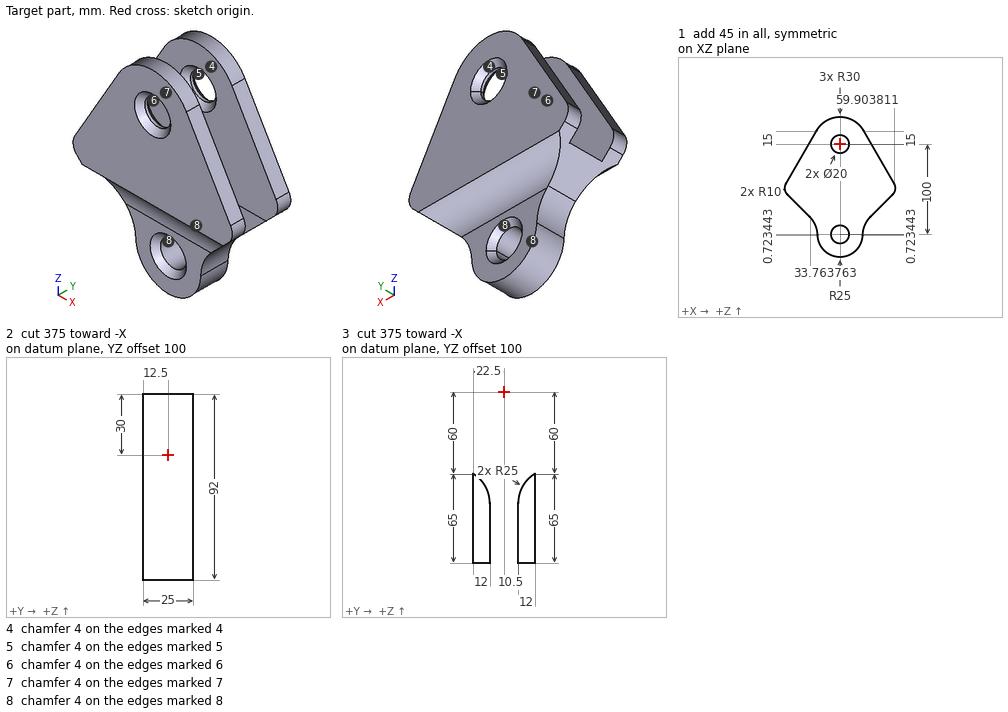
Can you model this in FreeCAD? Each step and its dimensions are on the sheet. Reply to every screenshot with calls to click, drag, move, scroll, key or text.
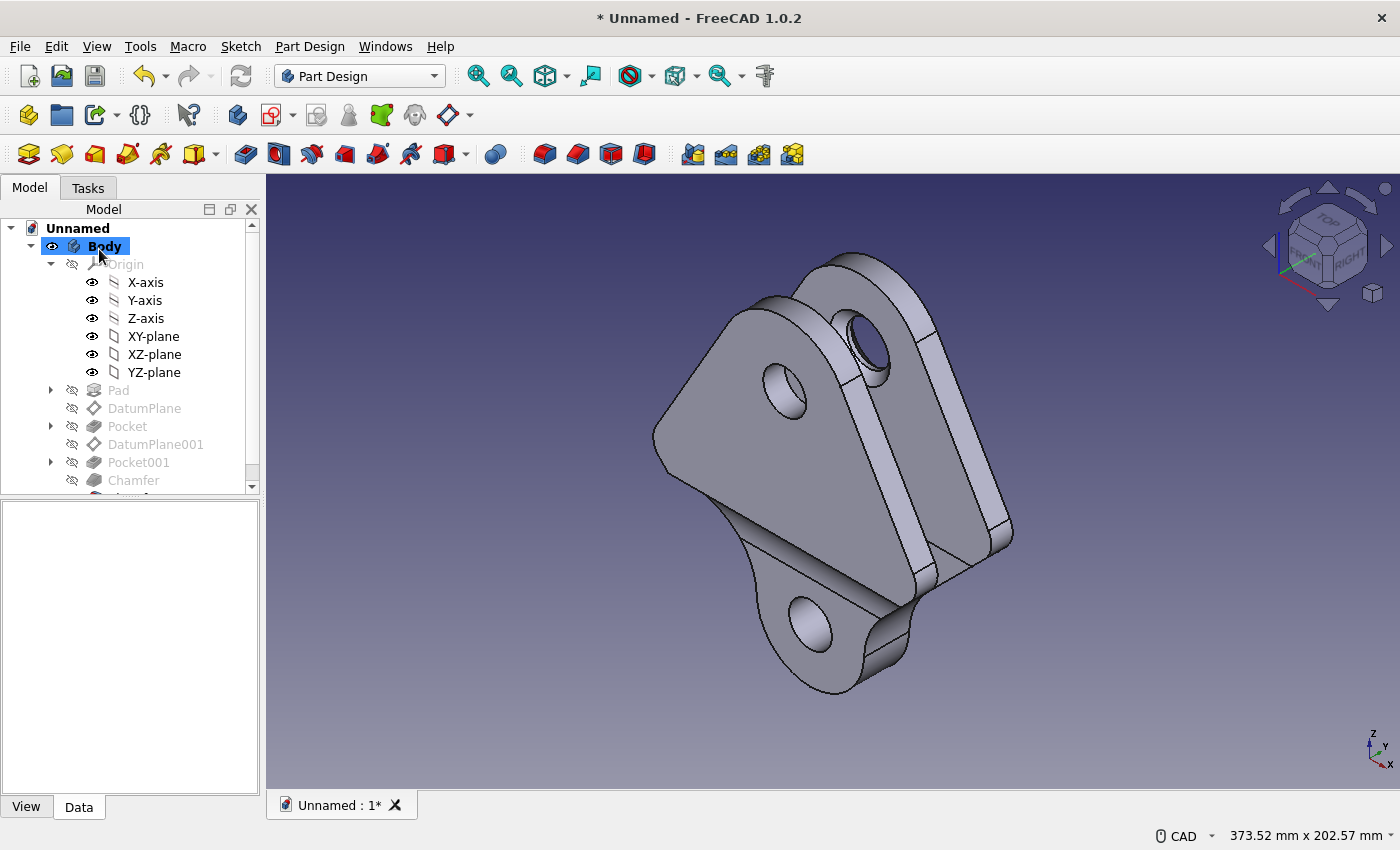
click(763, 378)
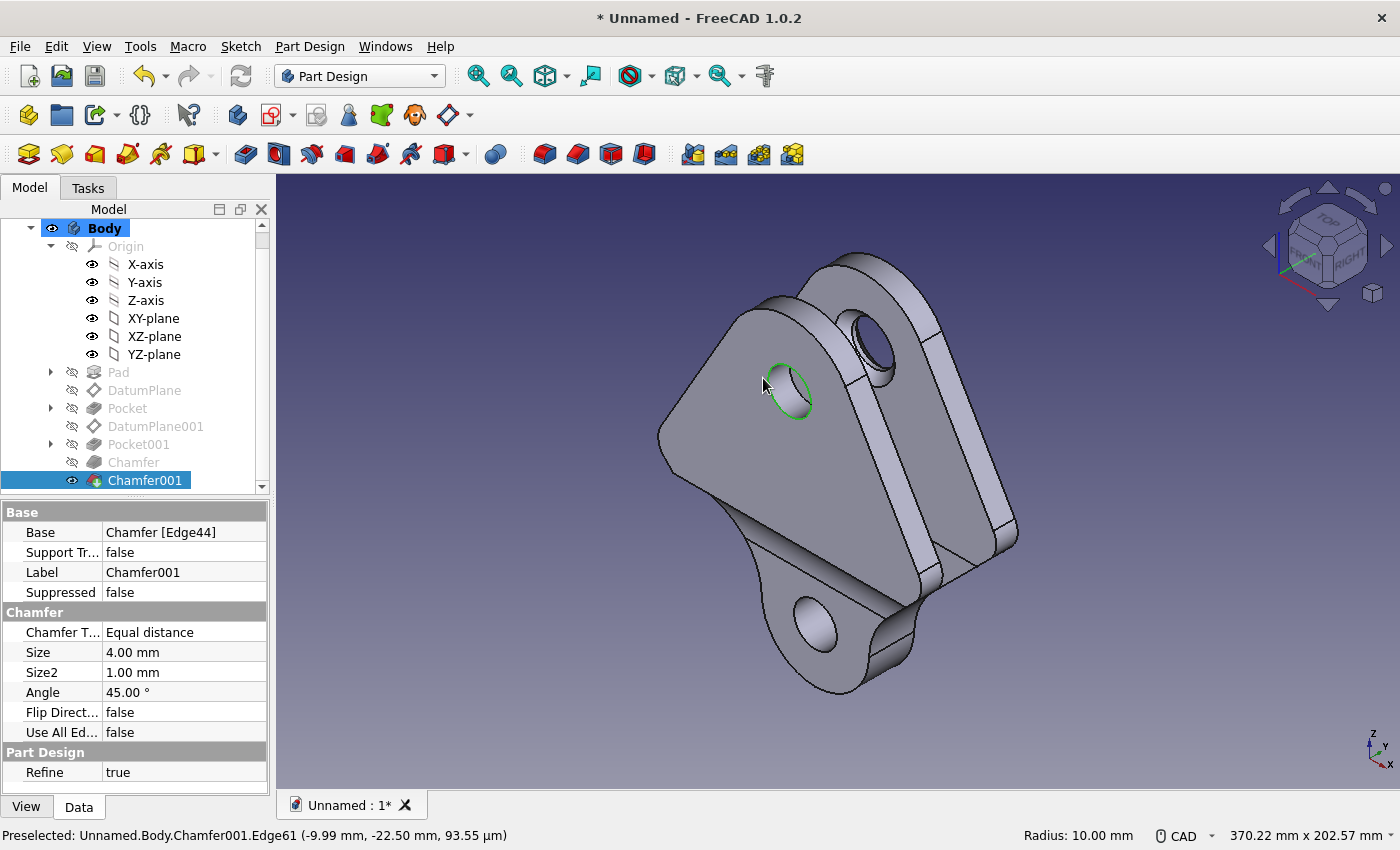
click(578, 154)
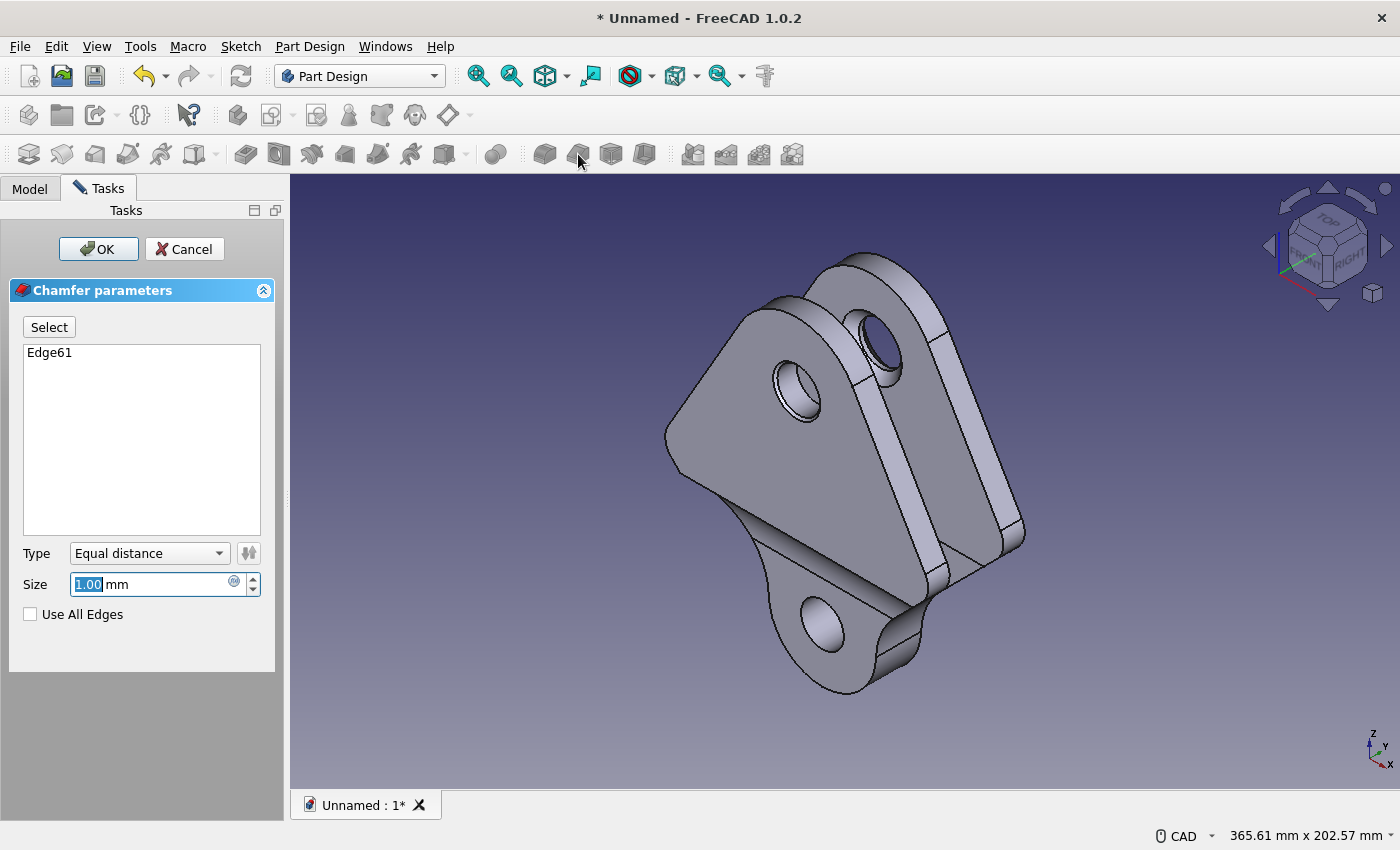
text(4)
key(Tab)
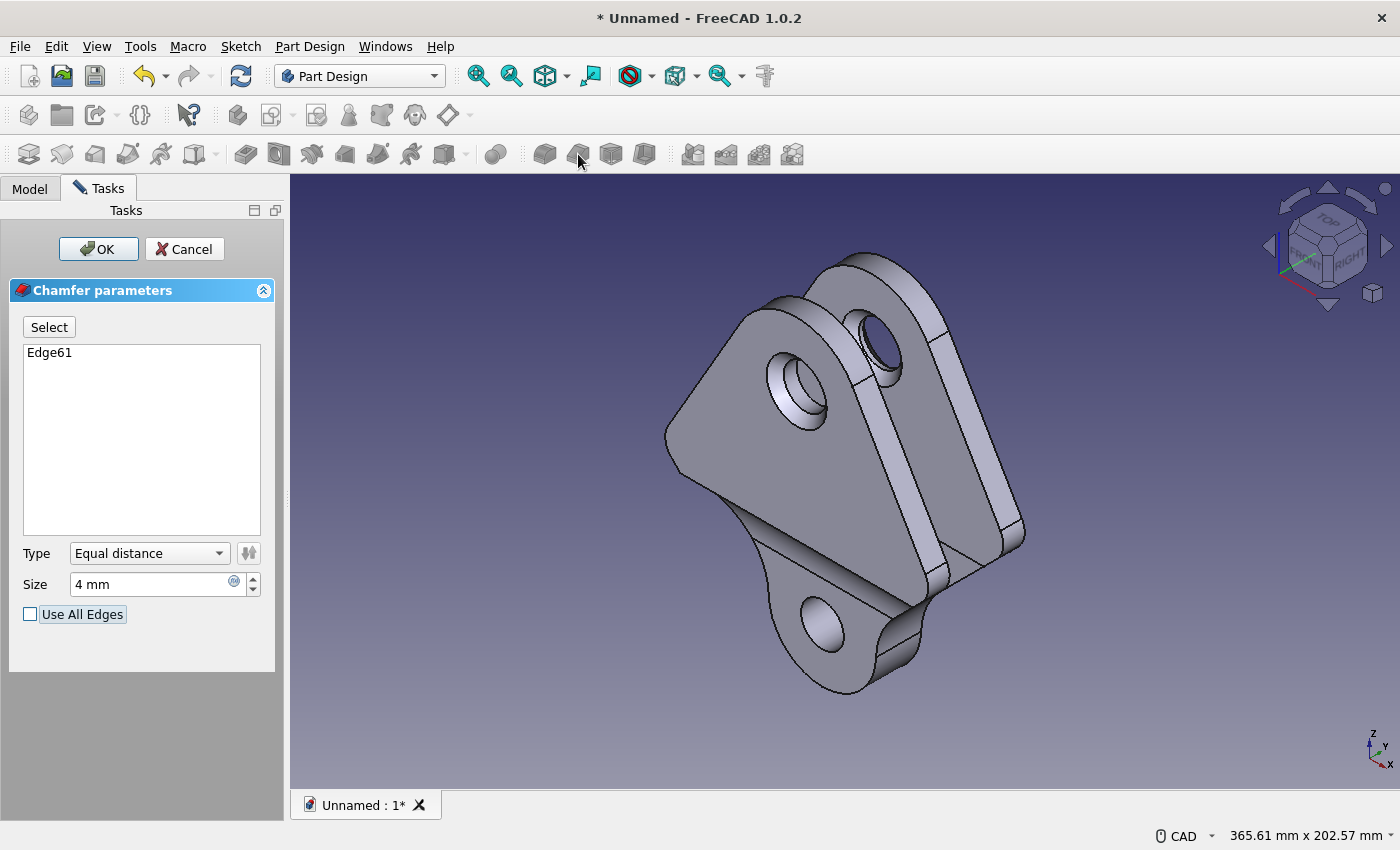
click(99, 249)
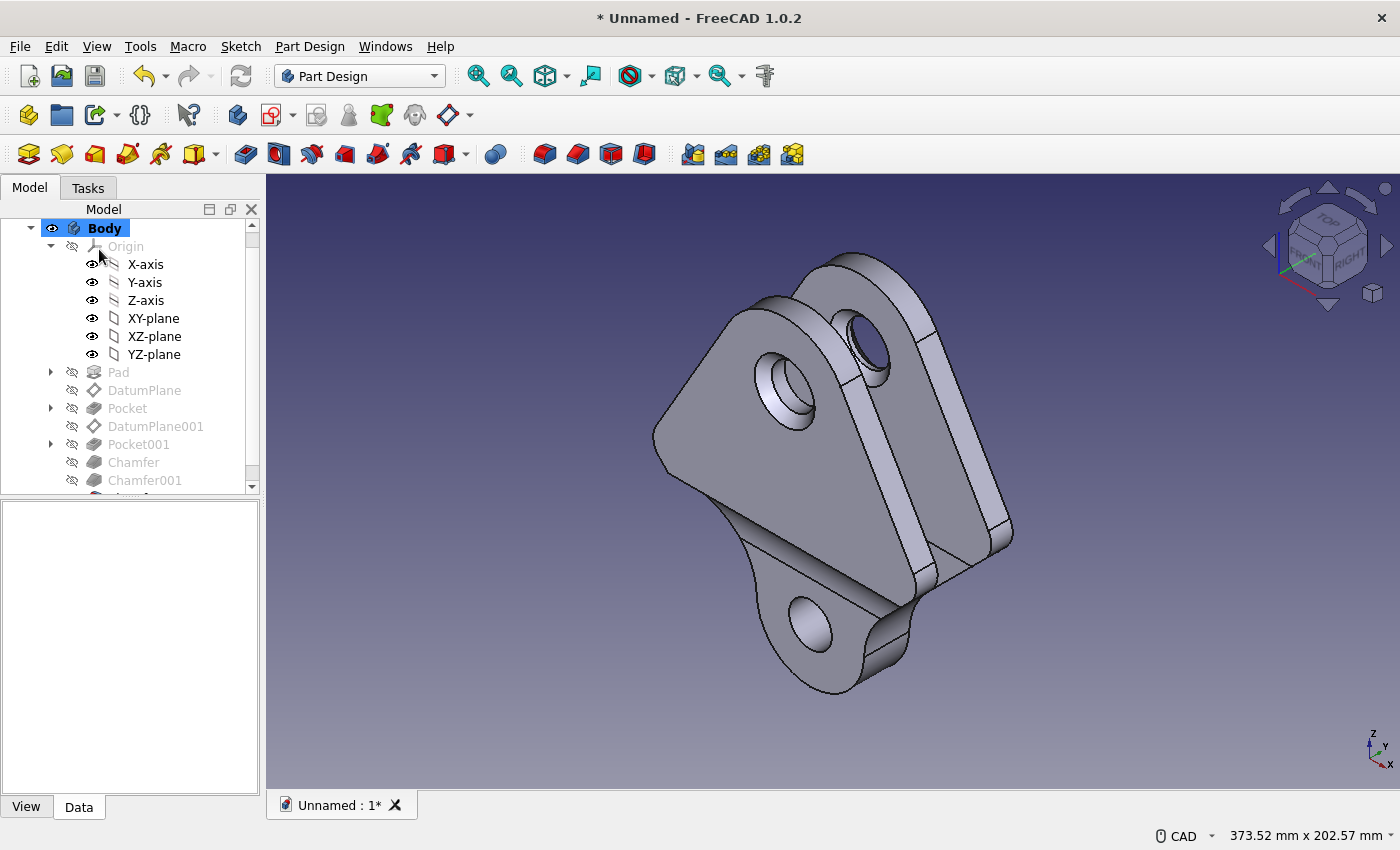
key(2)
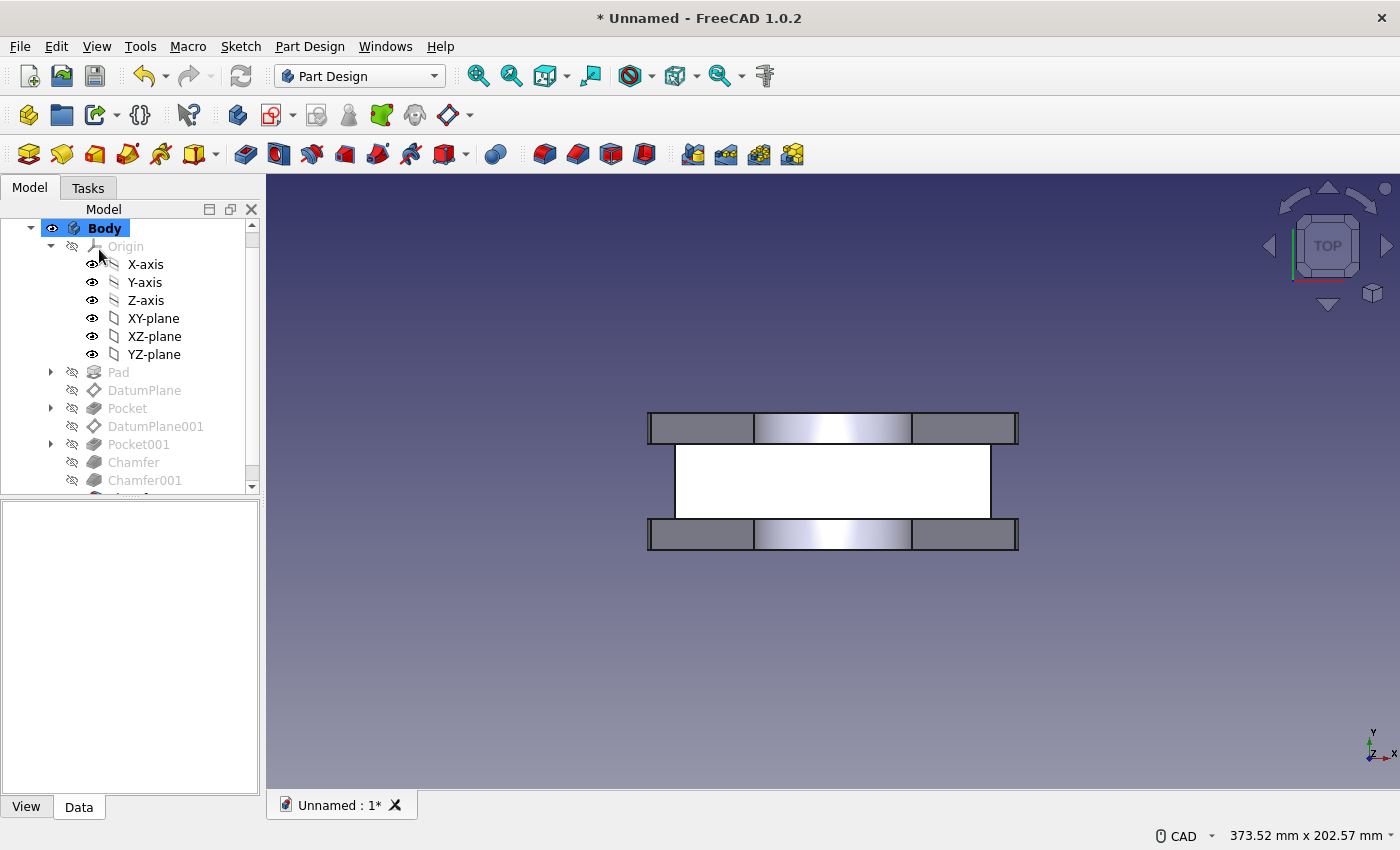
click(479, 76)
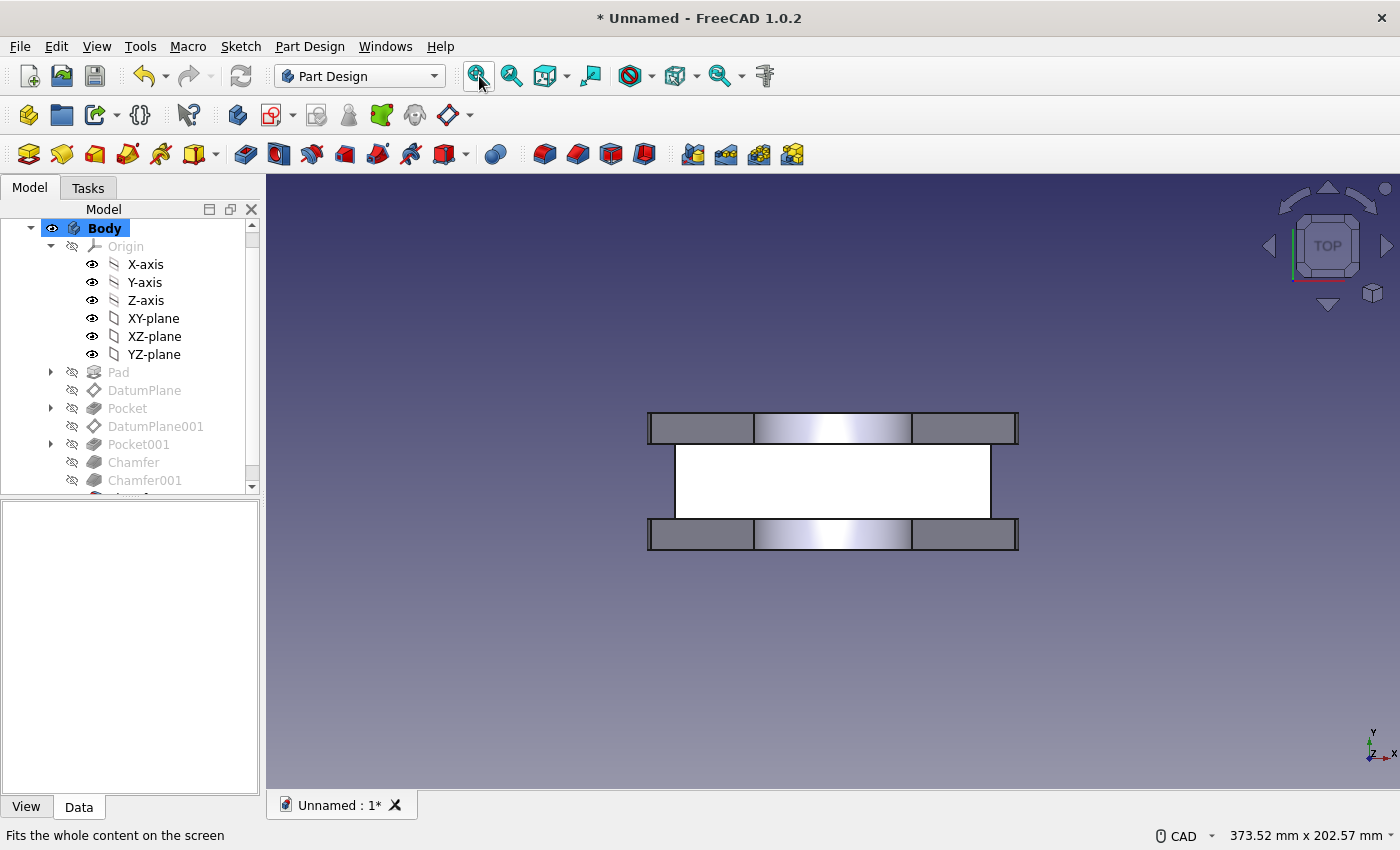
key(0)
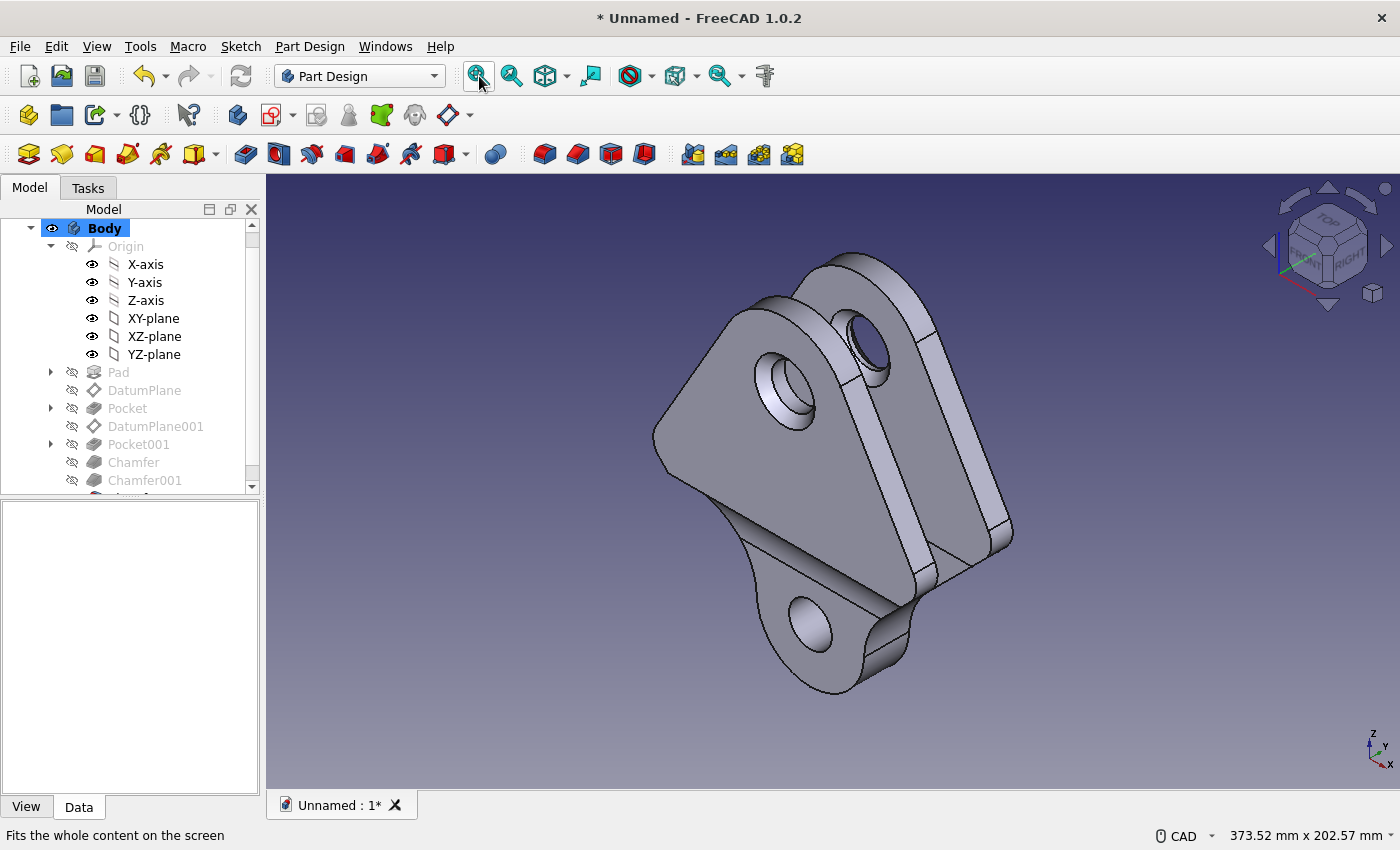
key(1)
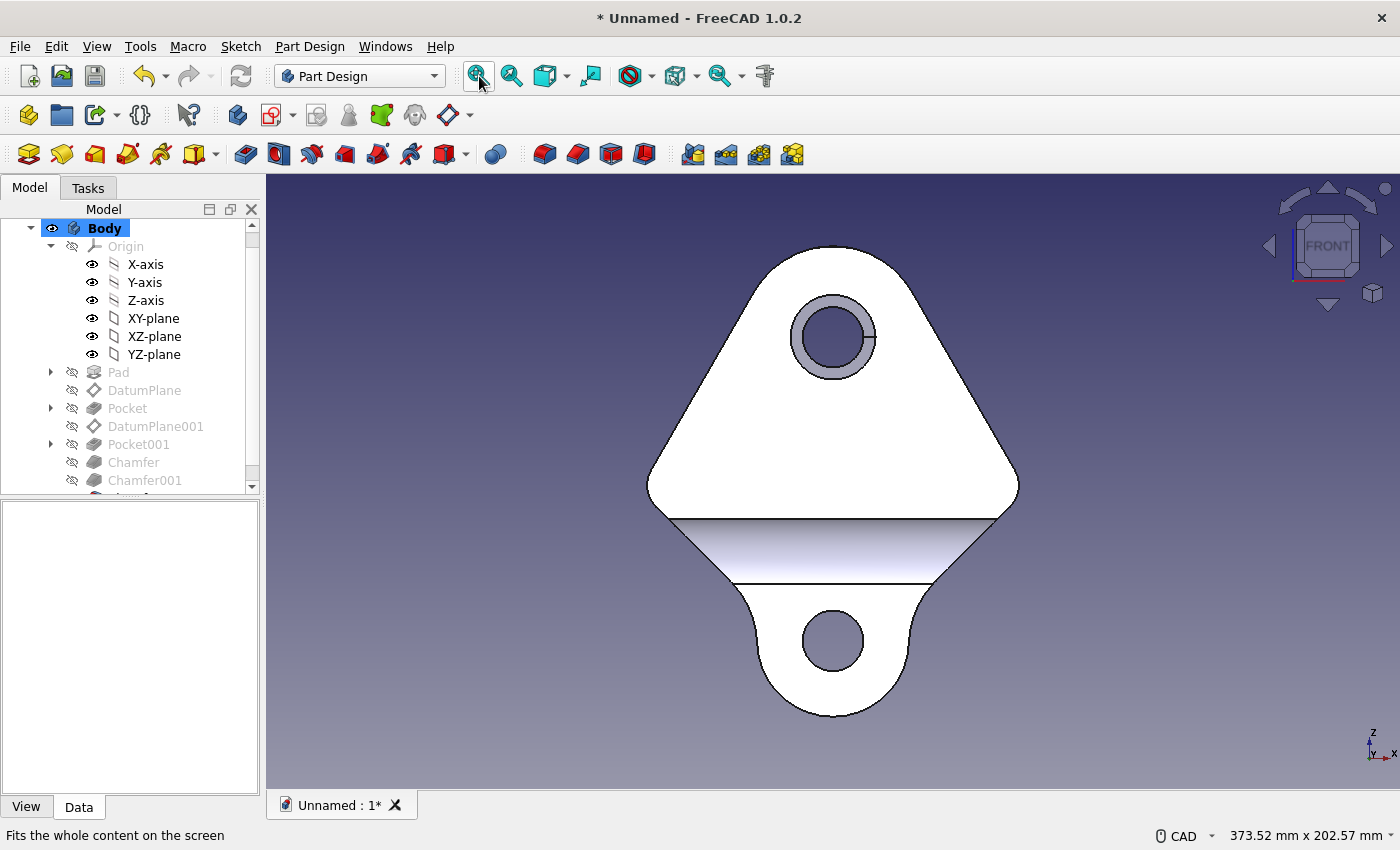
key(3)